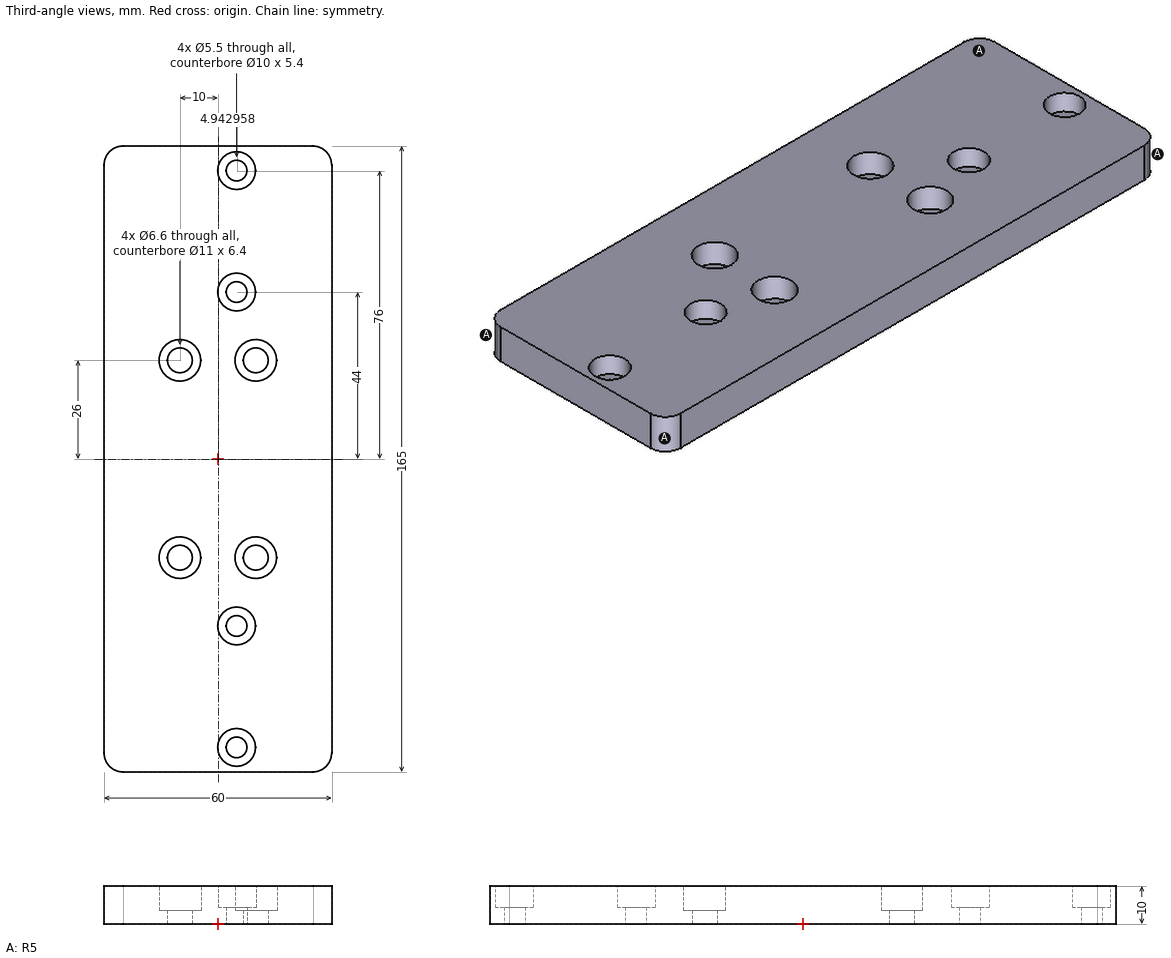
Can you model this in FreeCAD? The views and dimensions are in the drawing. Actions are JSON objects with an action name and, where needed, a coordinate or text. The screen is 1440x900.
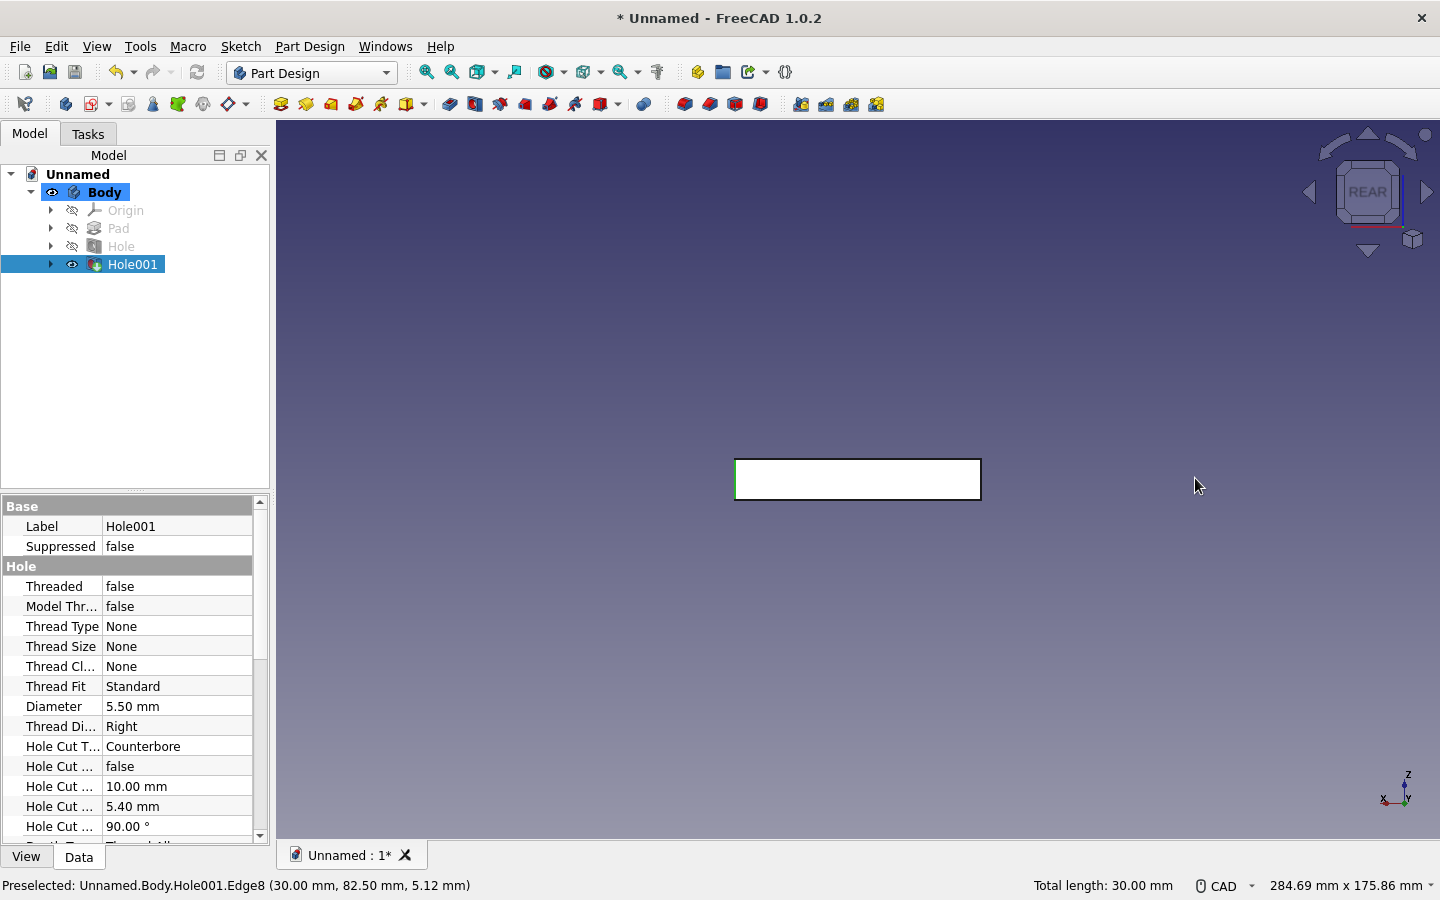
{"action": "left_click", "coordinate": [427, 72]}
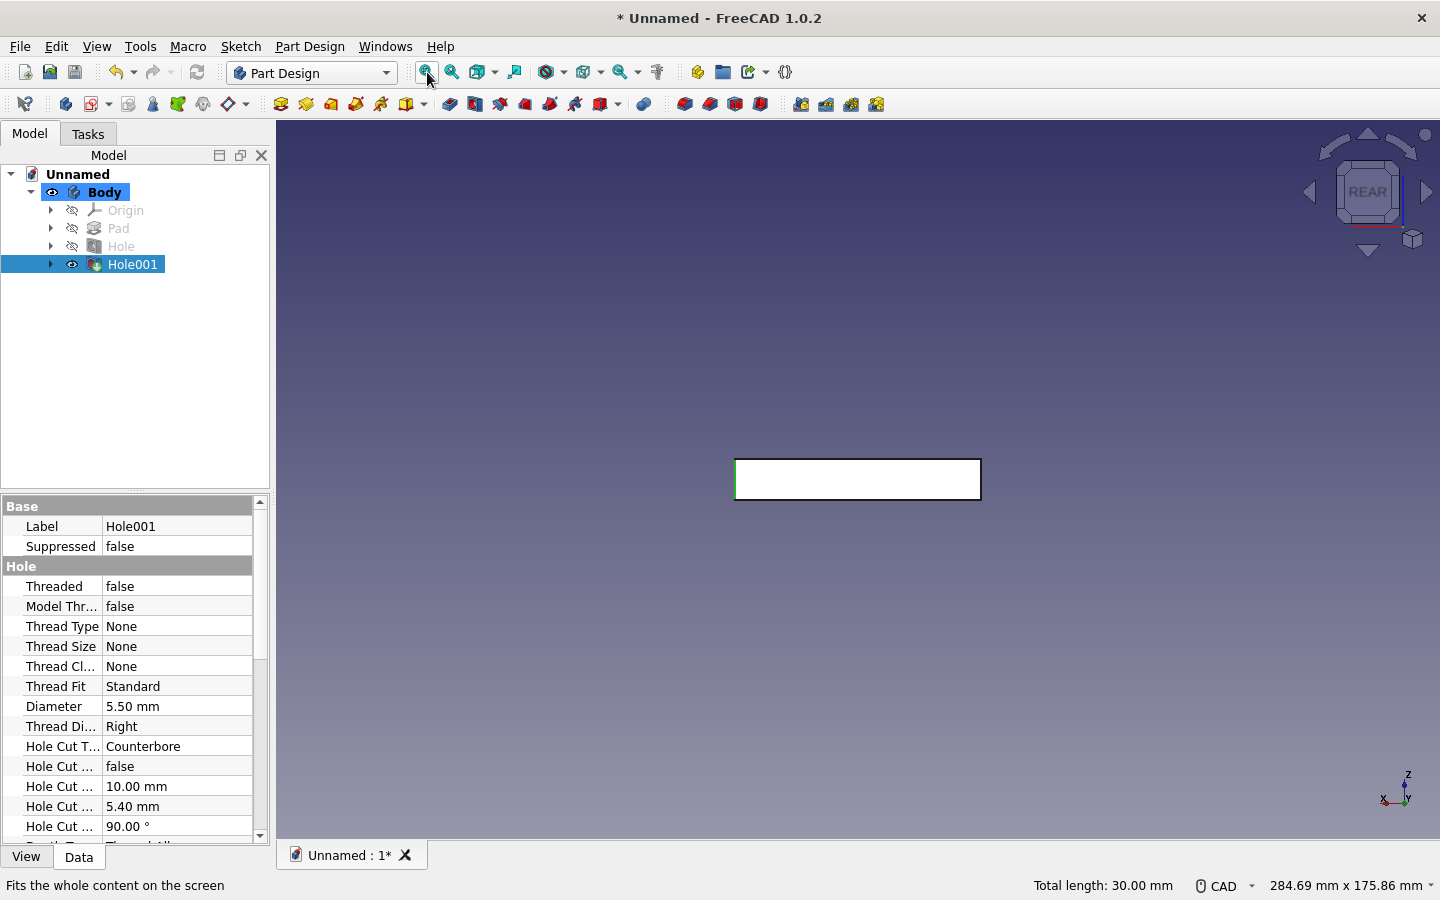
{"action": "left_click", "coordinate": [981, 479], "text": "ctrl"}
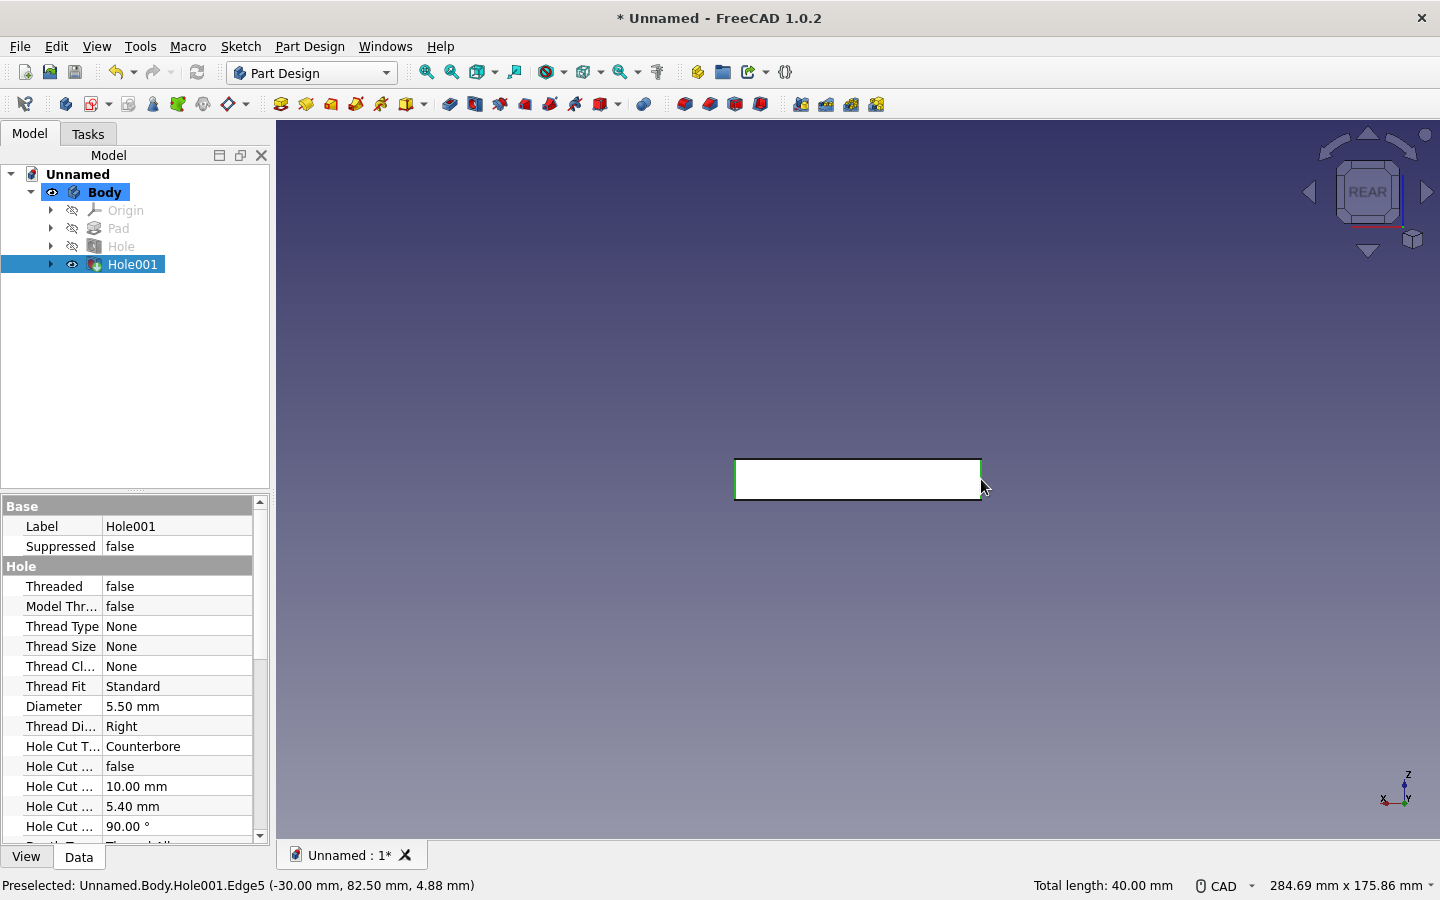
{"action": "left_click", "coordinate": [685, 104]}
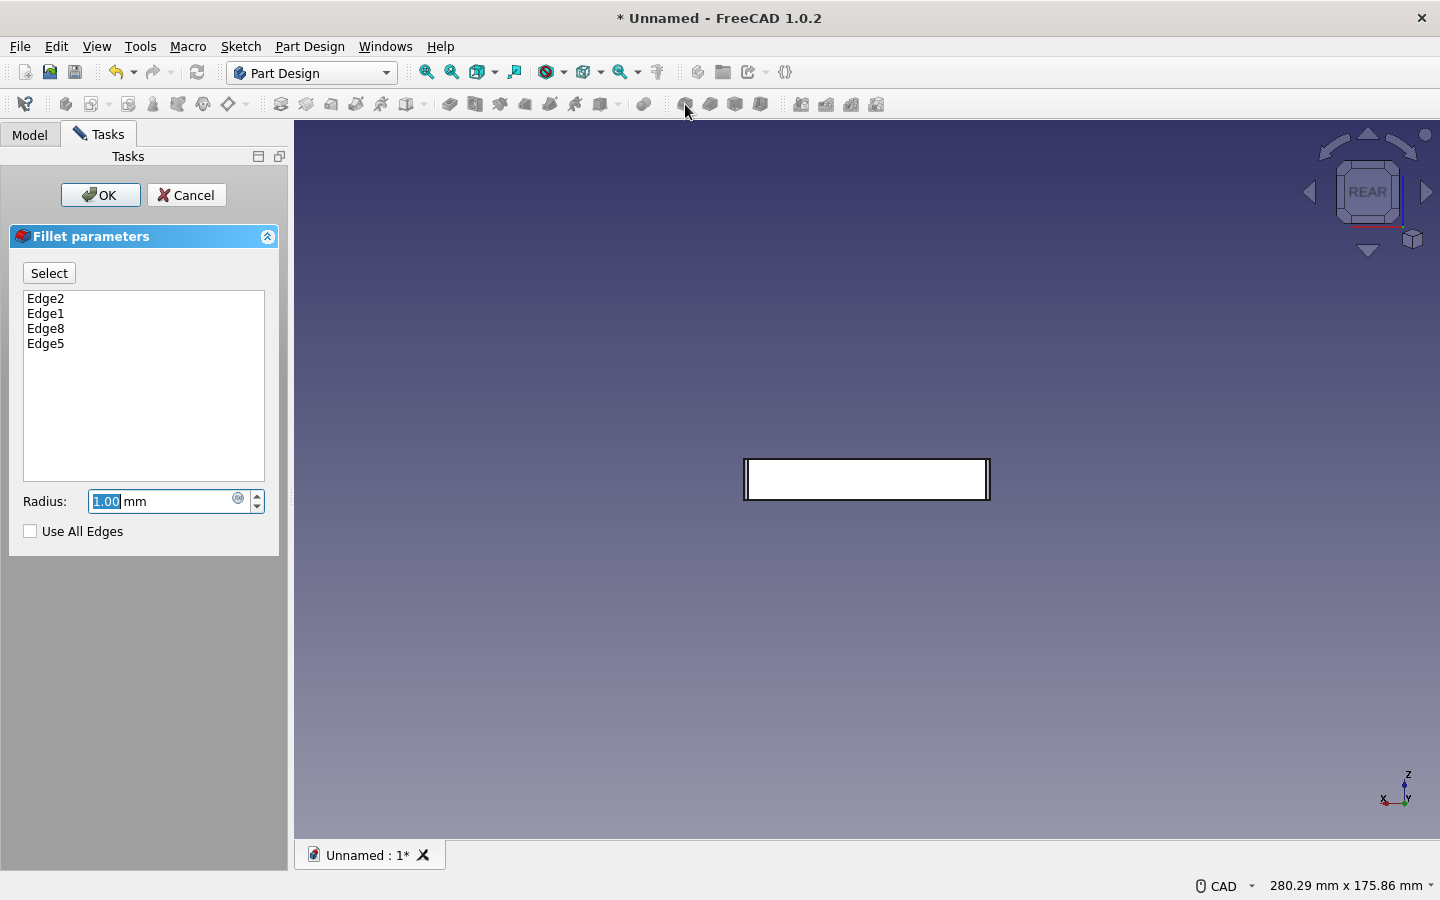
{"action": "type", "text": "5"}
{"action": "key", "text": "Tab"}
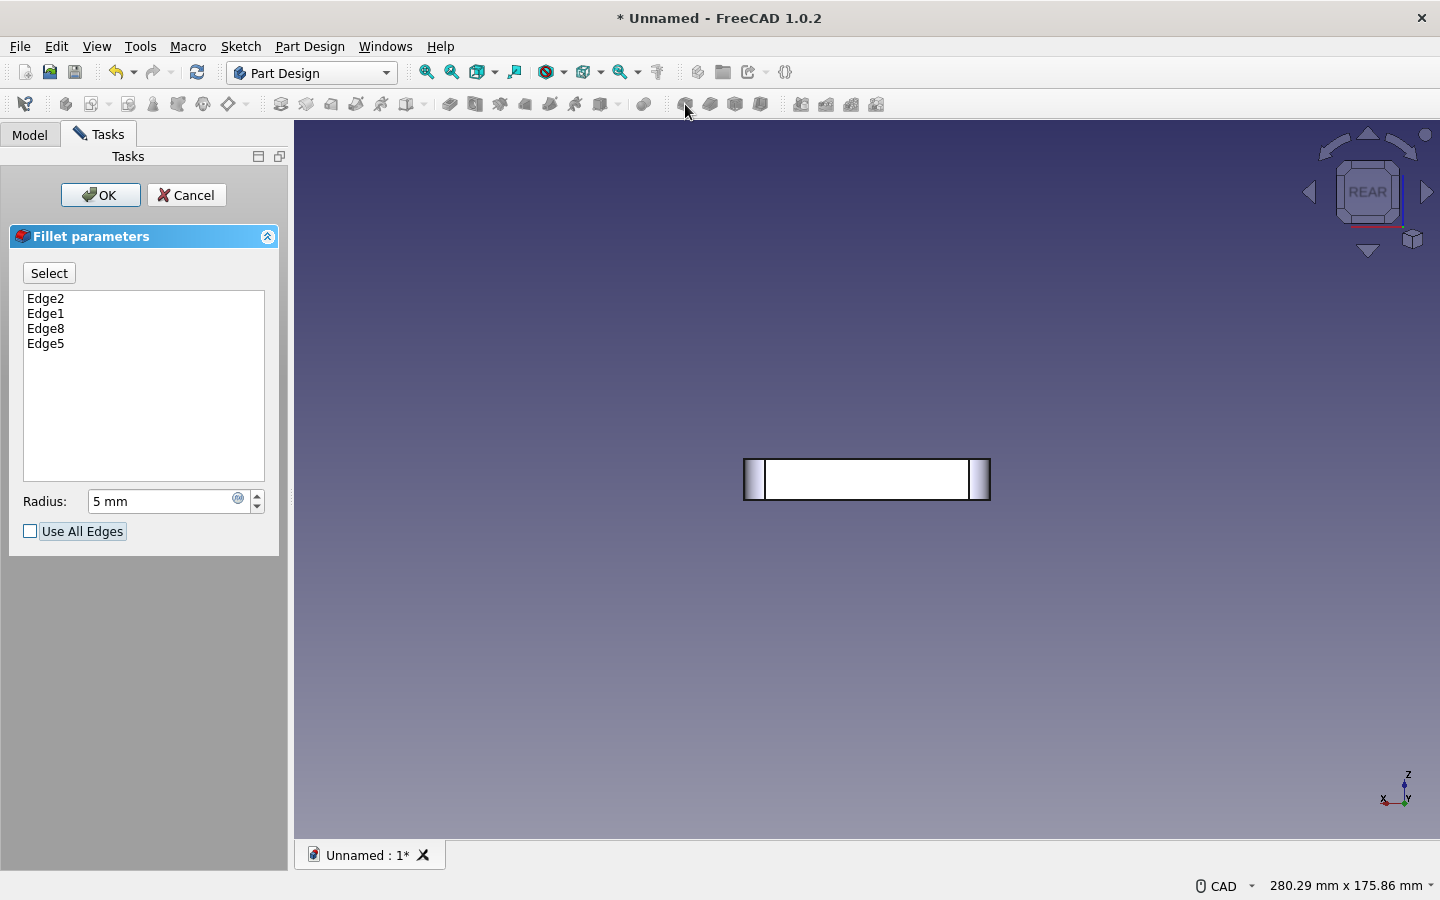
{"action": "left_click", "coordinate": [101, 195]}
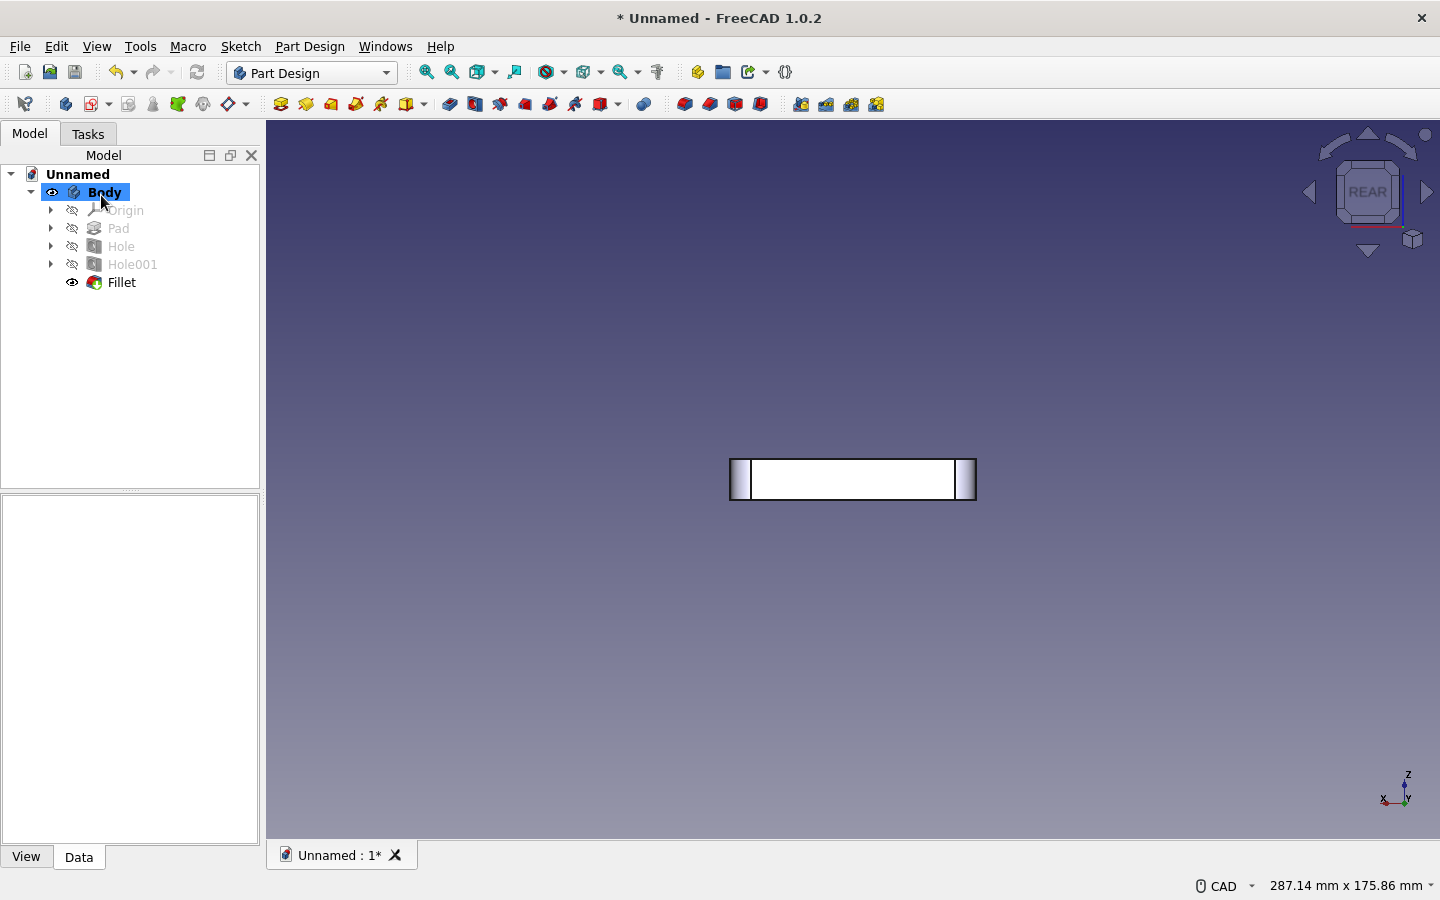
{"action": "key", "text": "0"}